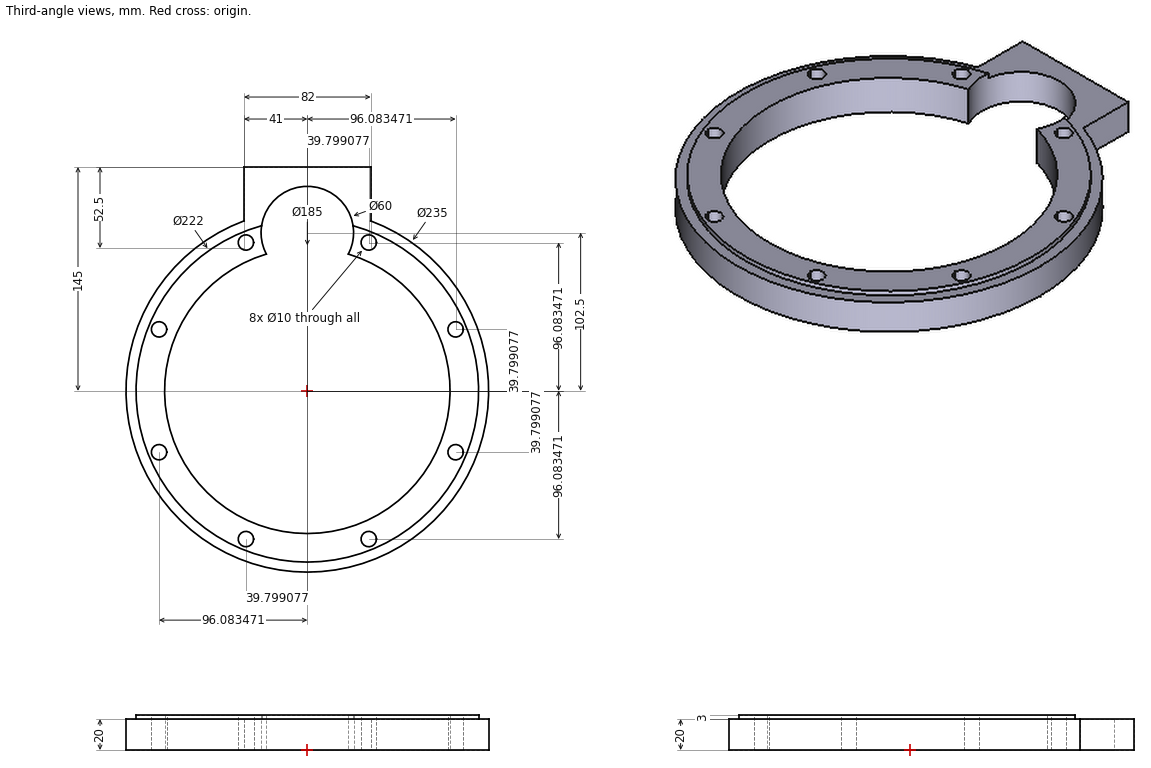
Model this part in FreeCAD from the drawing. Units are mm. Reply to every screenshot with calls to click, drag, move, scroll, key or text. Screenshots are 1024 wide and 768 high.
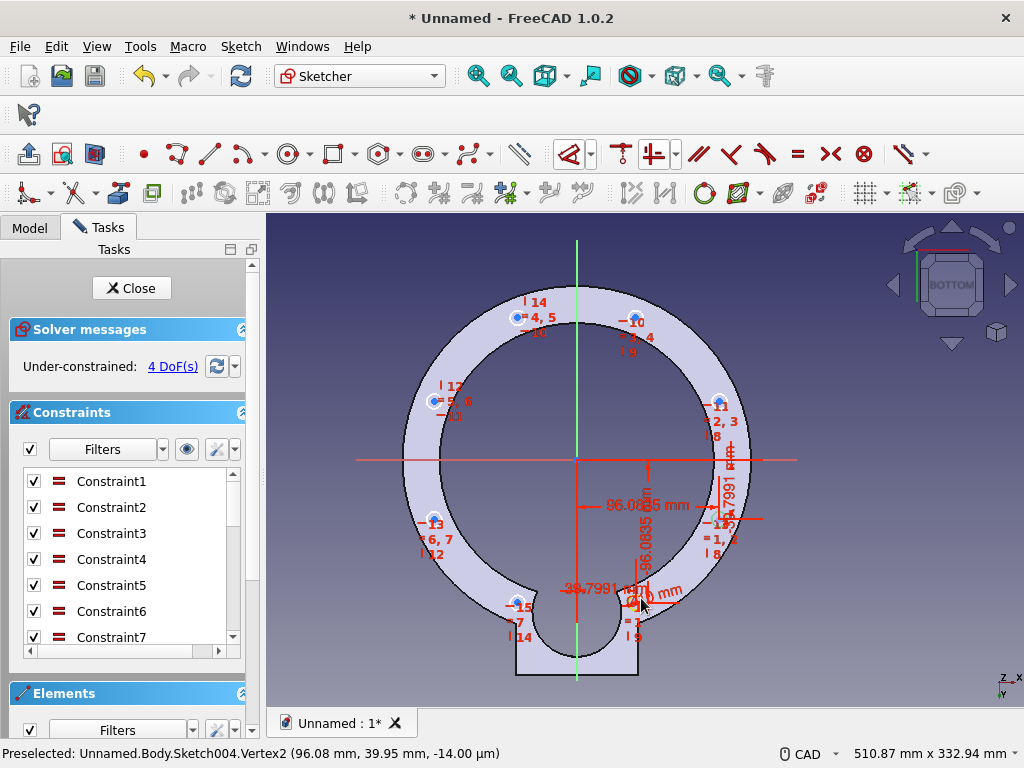
click(719, 401)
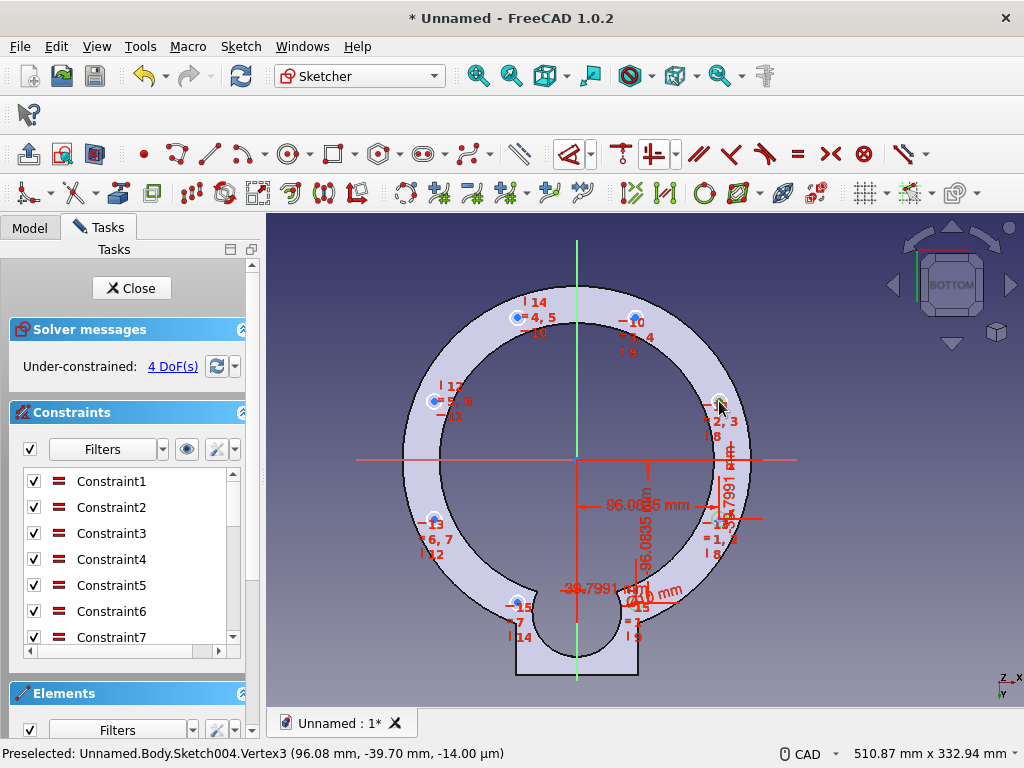
key(i)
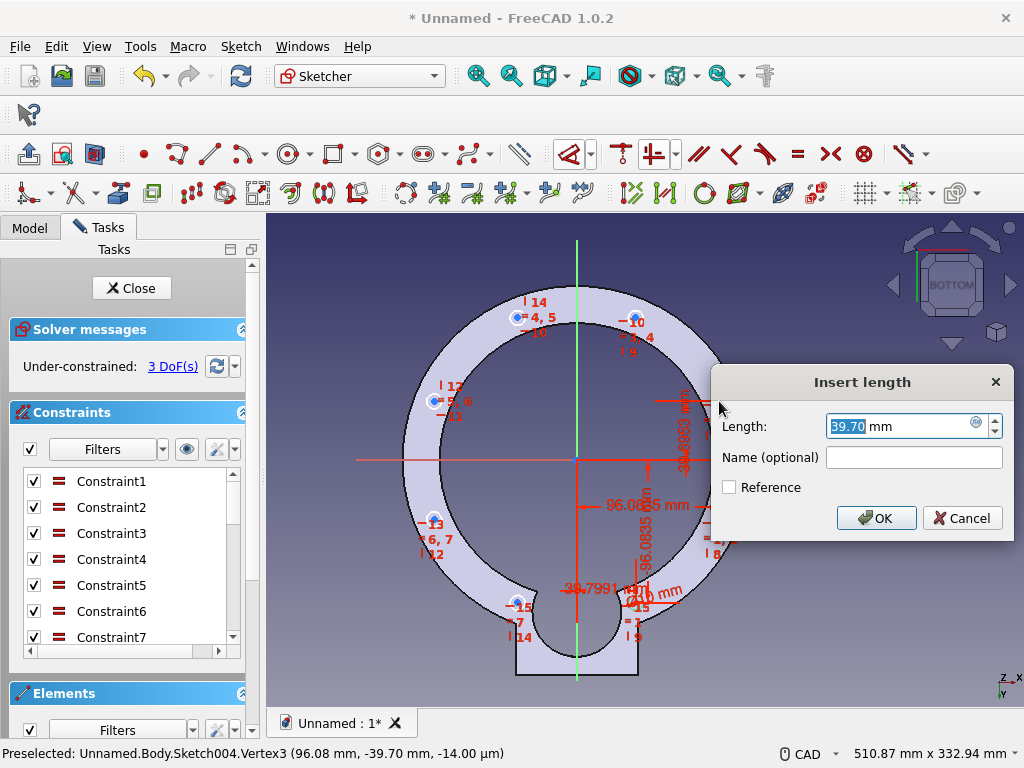
text(39.799077)
key(Return)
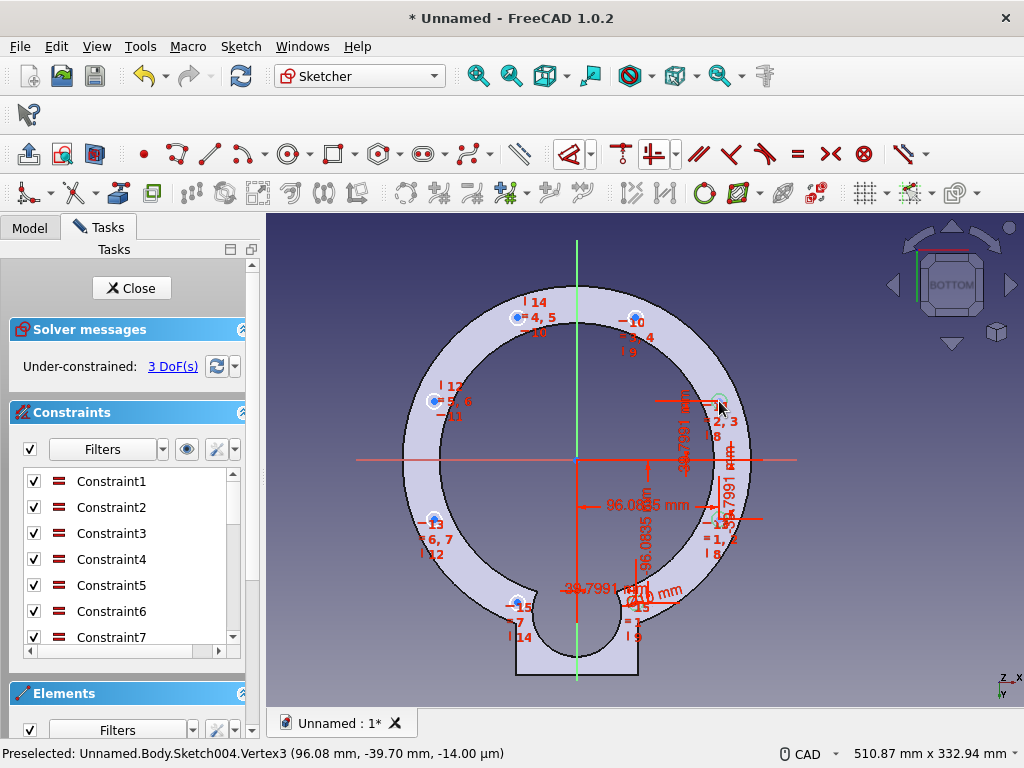
click(636, 318)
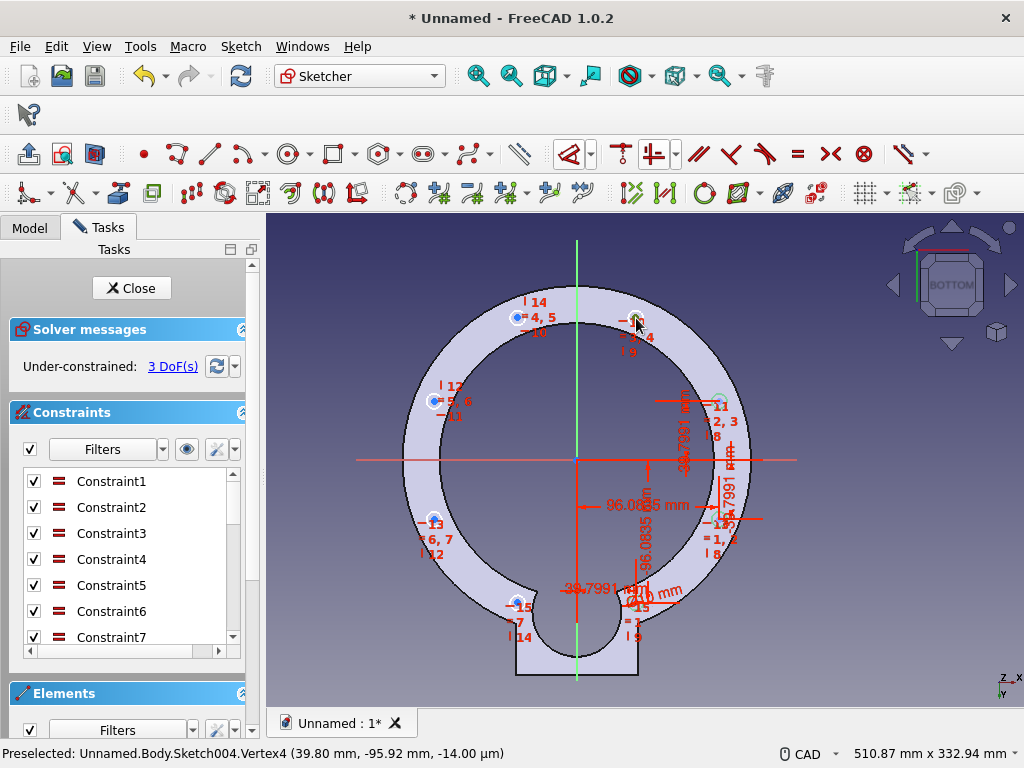
click(590, 154)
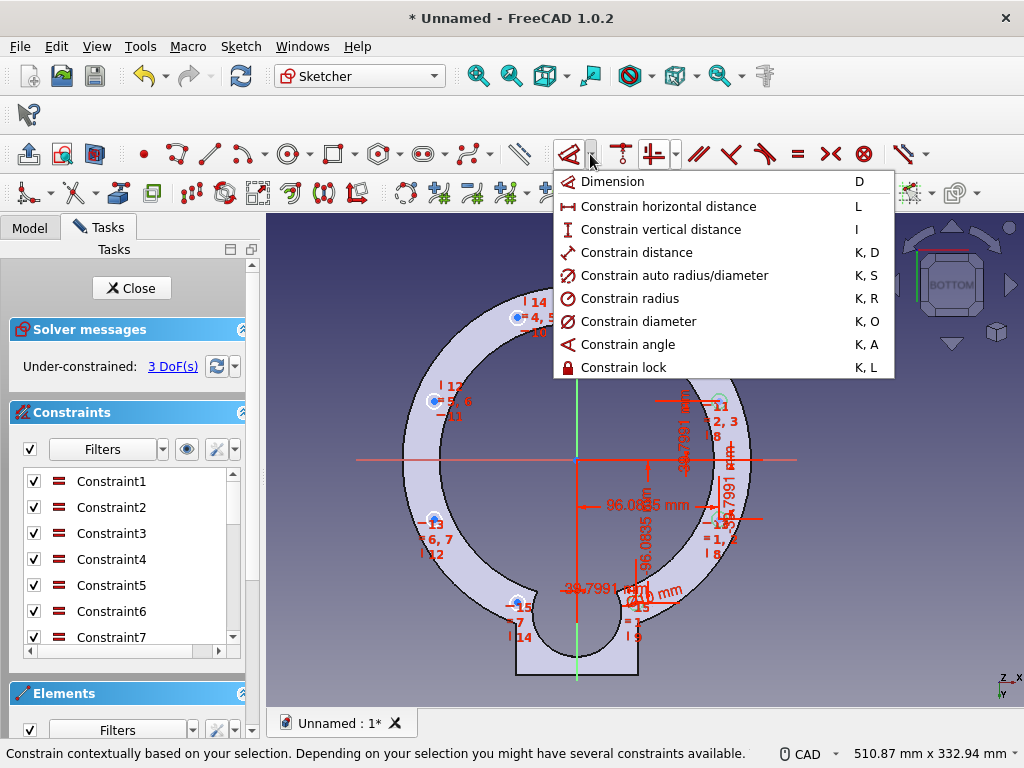
click(724, 230)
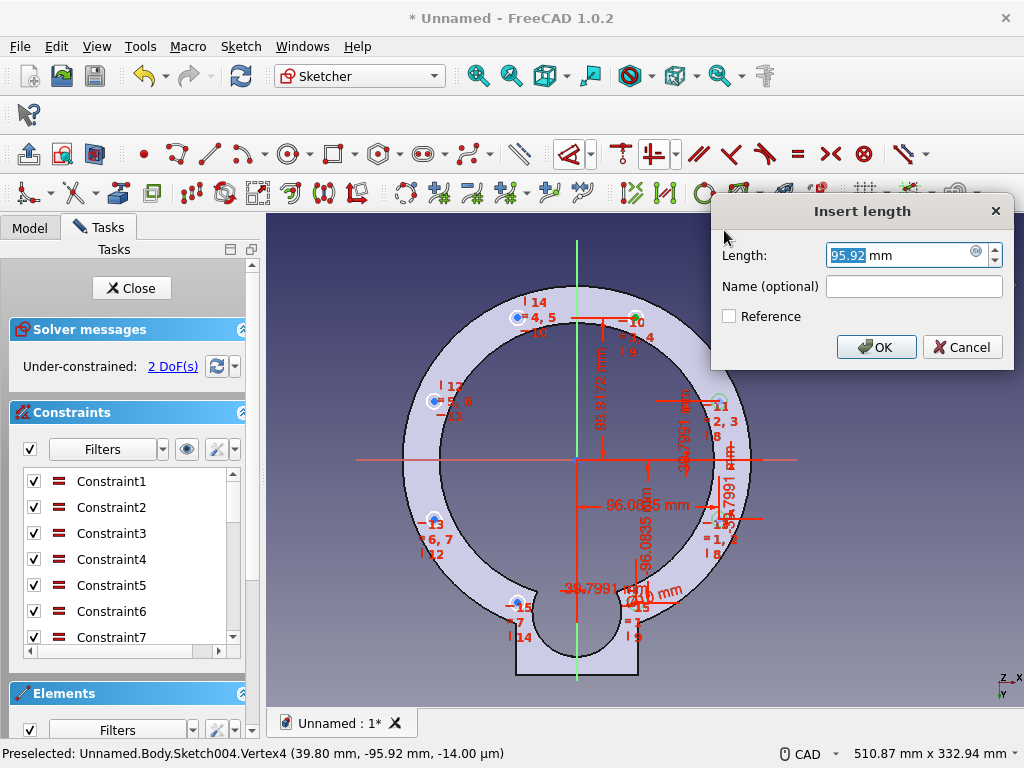
text(96.083471)
key(Return)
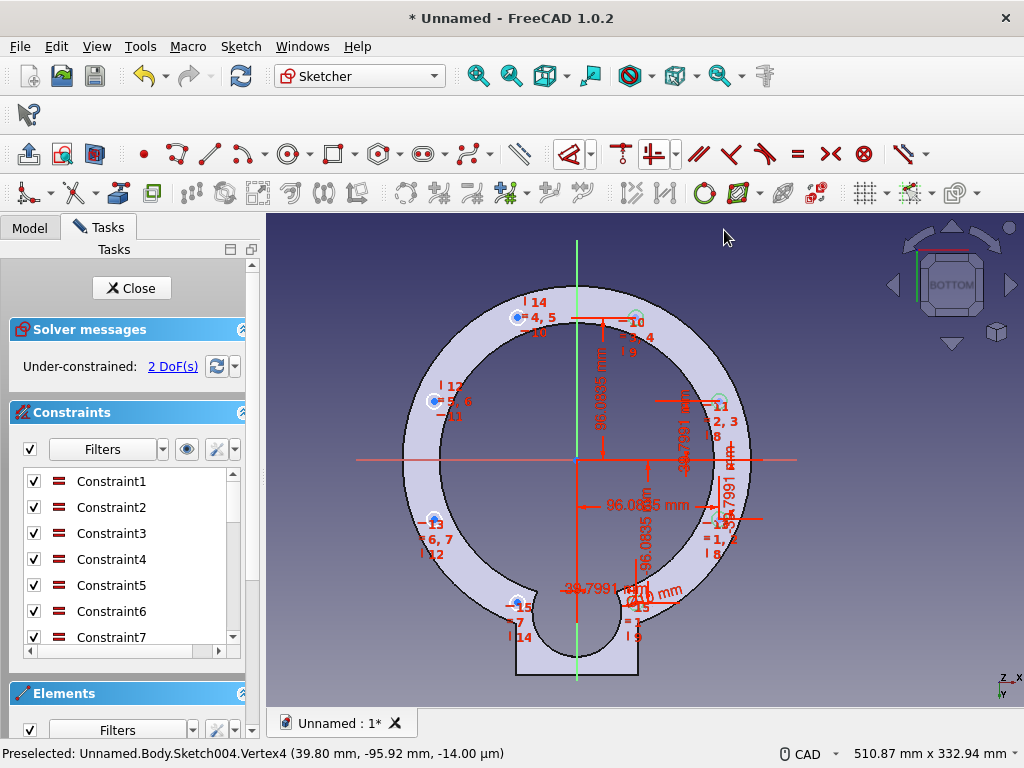
click(518, 318)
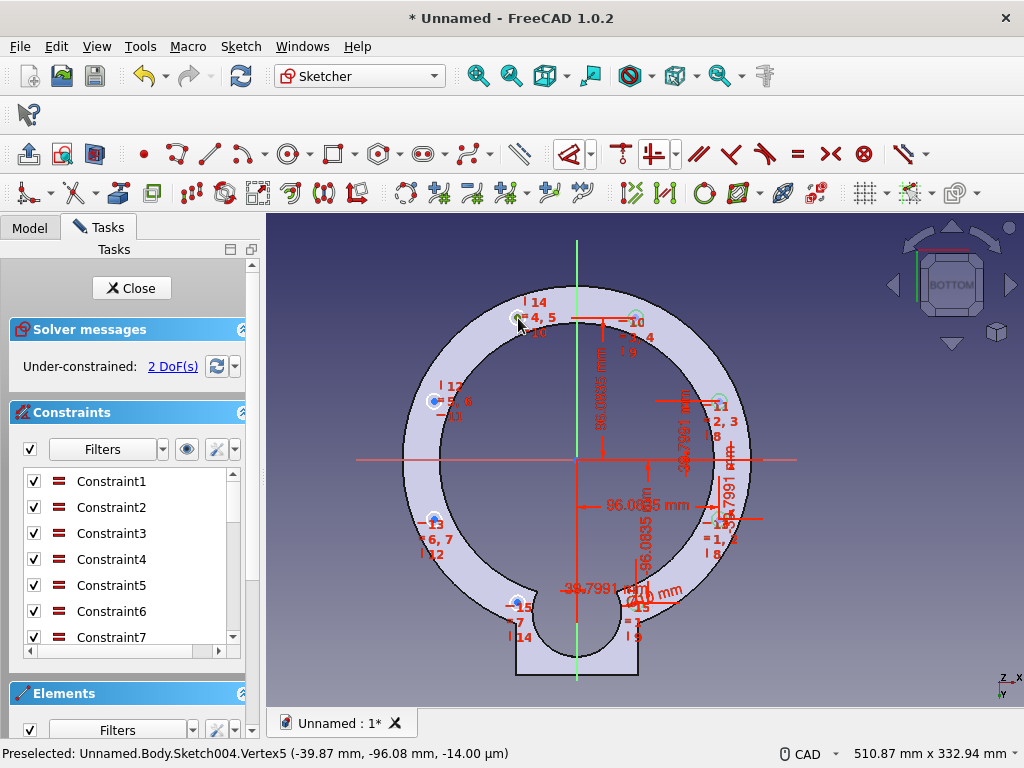
click(590, 154)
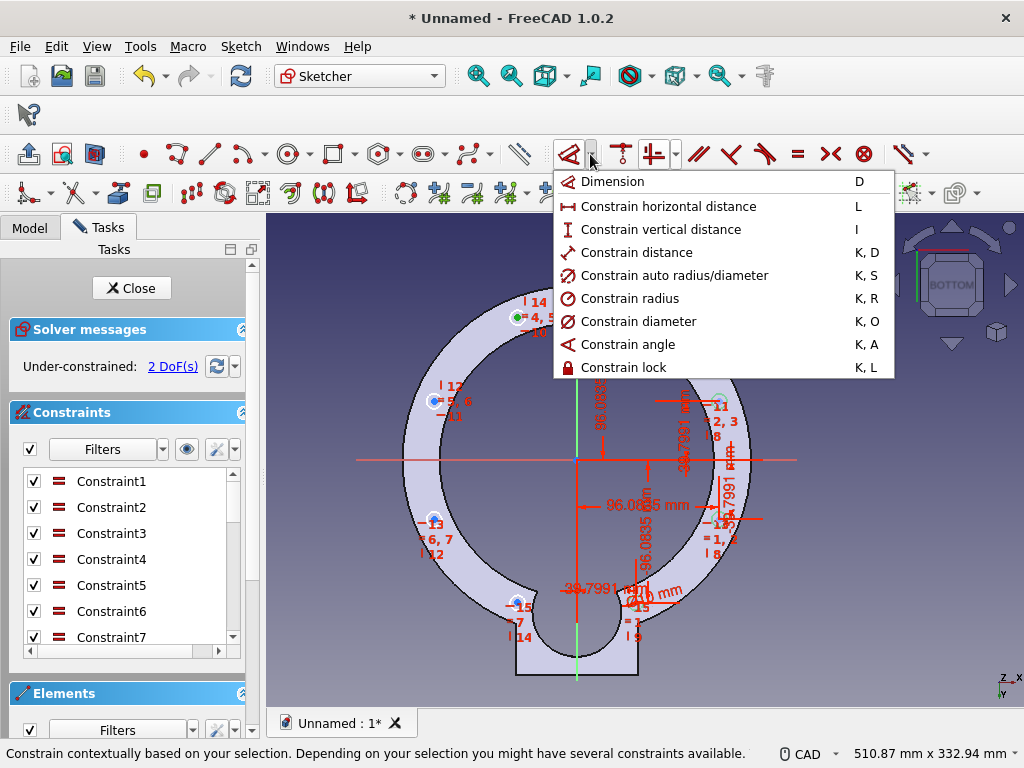
click(724, 206)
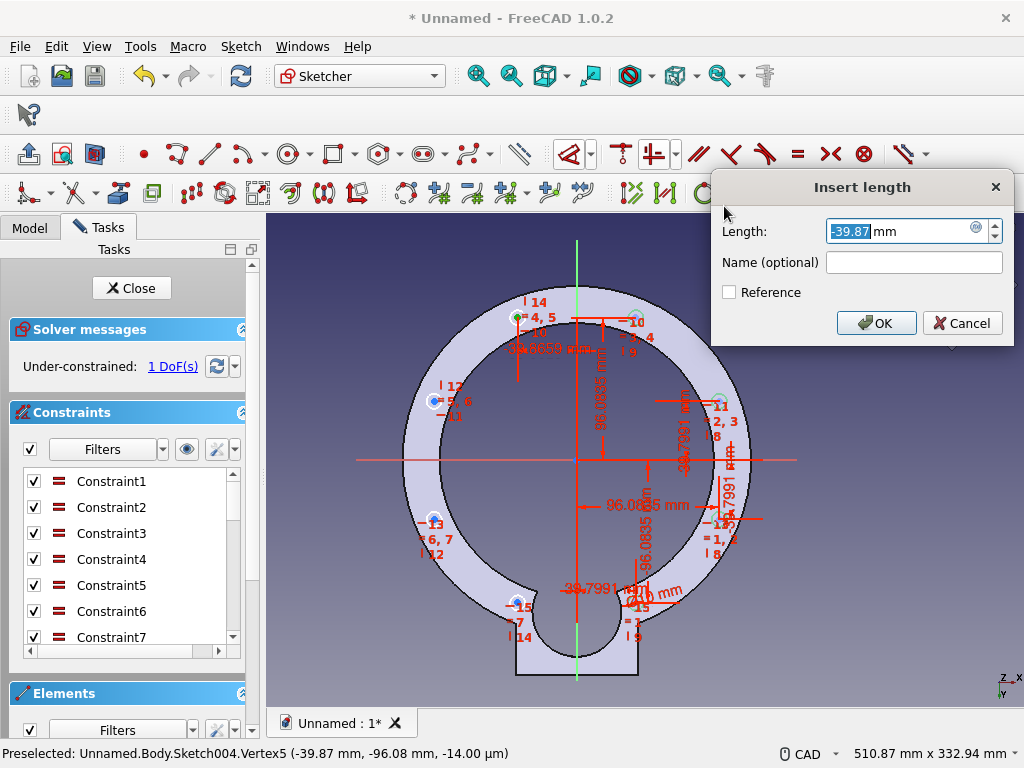
text(-39.799077)
key(Return)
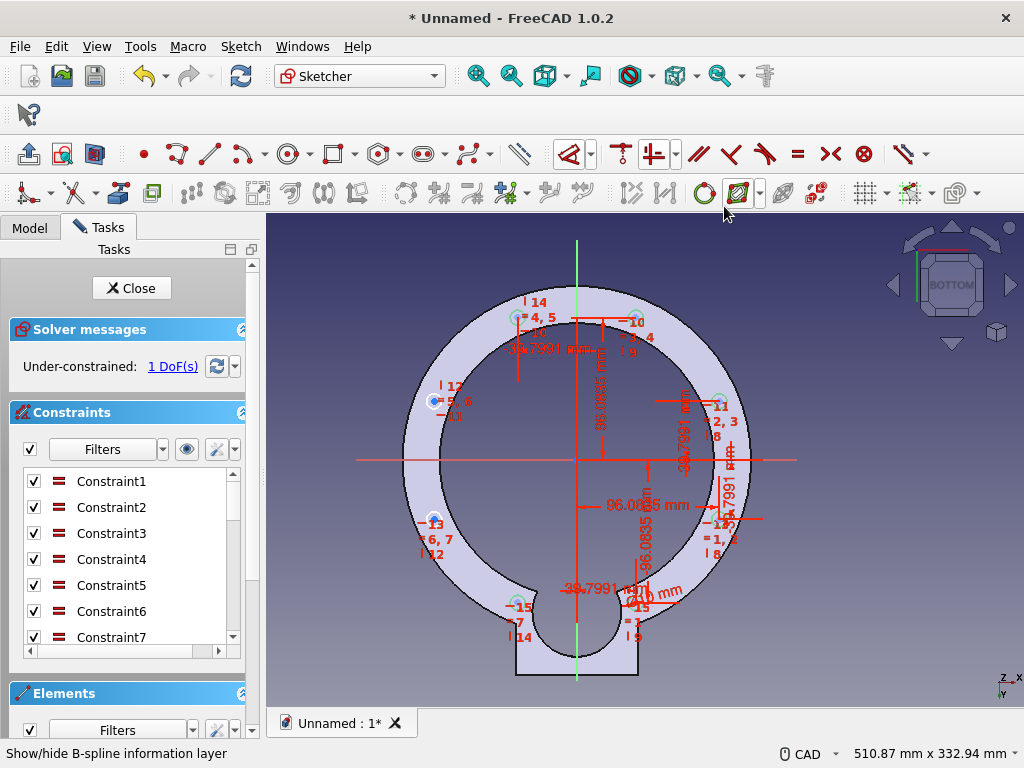
click(434, 401)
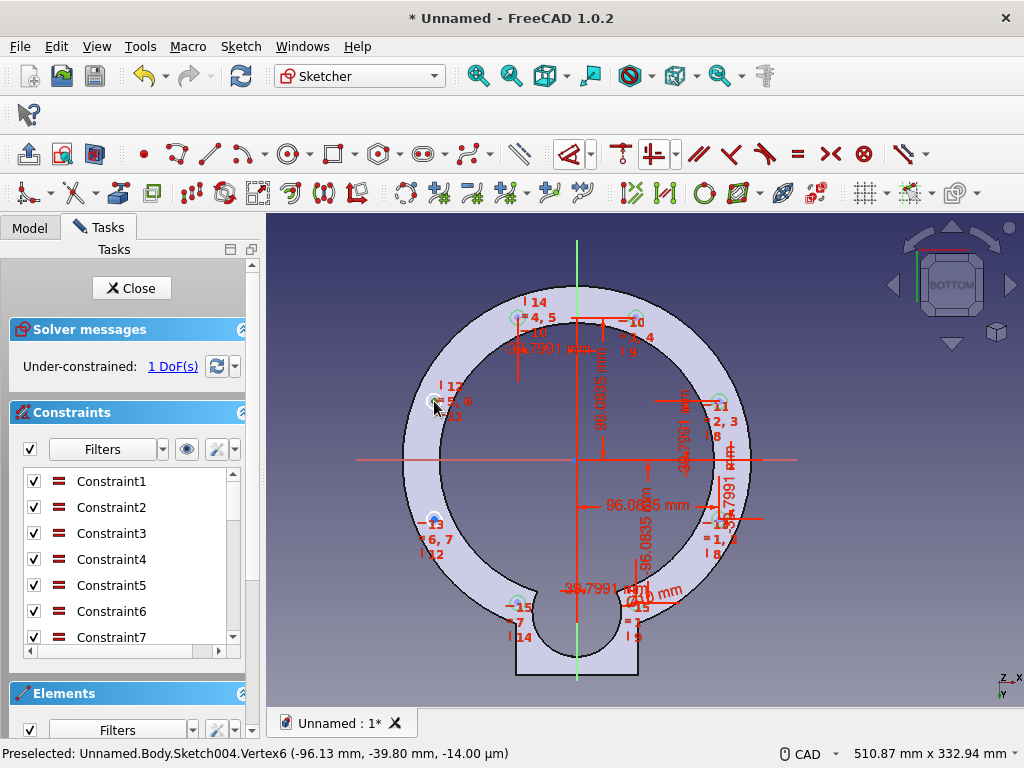
click(590, 154)